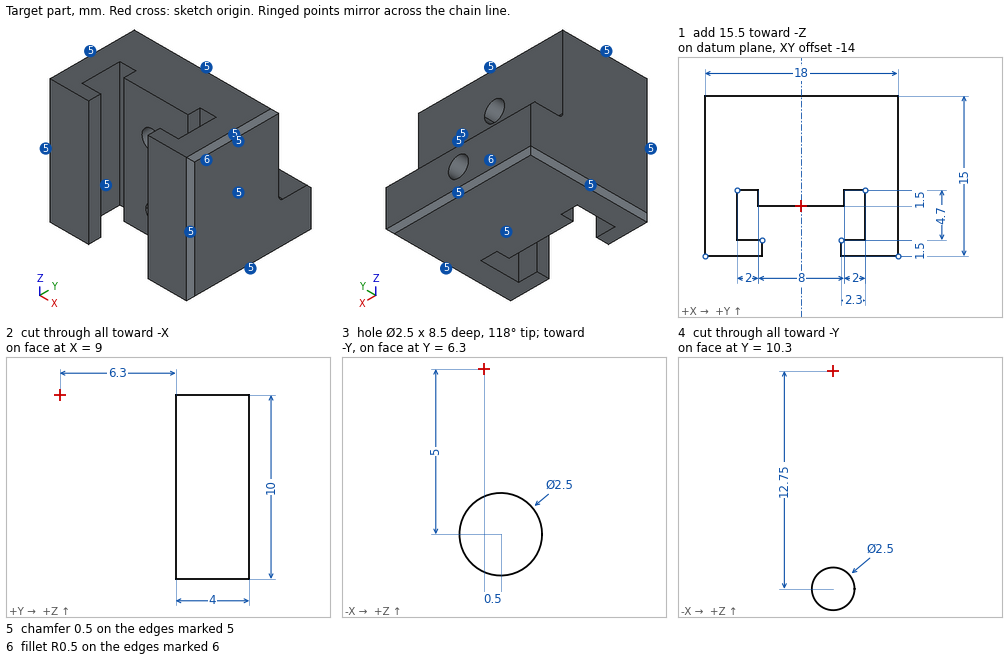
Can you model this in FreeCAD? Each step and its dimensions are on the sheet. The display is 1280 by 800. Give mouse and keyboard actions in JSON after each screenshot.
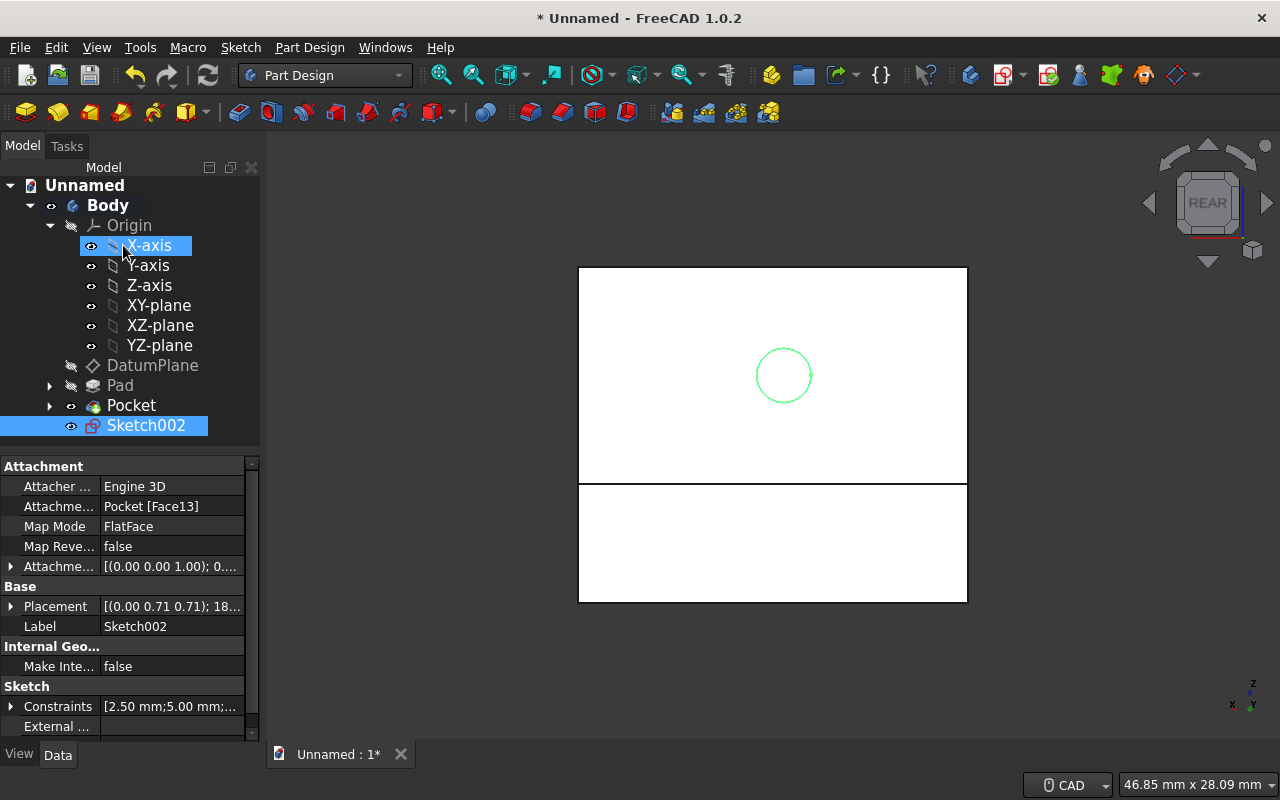
{"action": "left_click", "coordinate": [272, 112]}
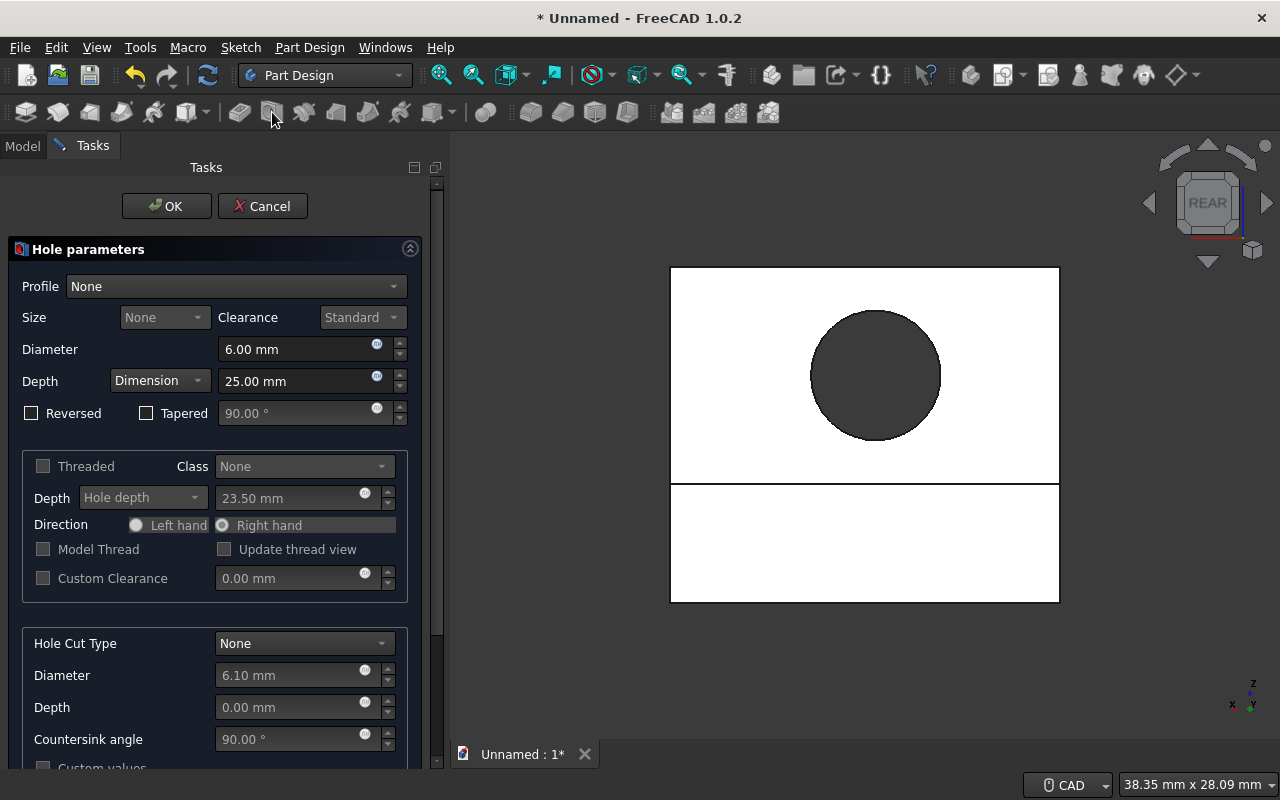
{"action": "triple_click", "coordinate": [305, 349]}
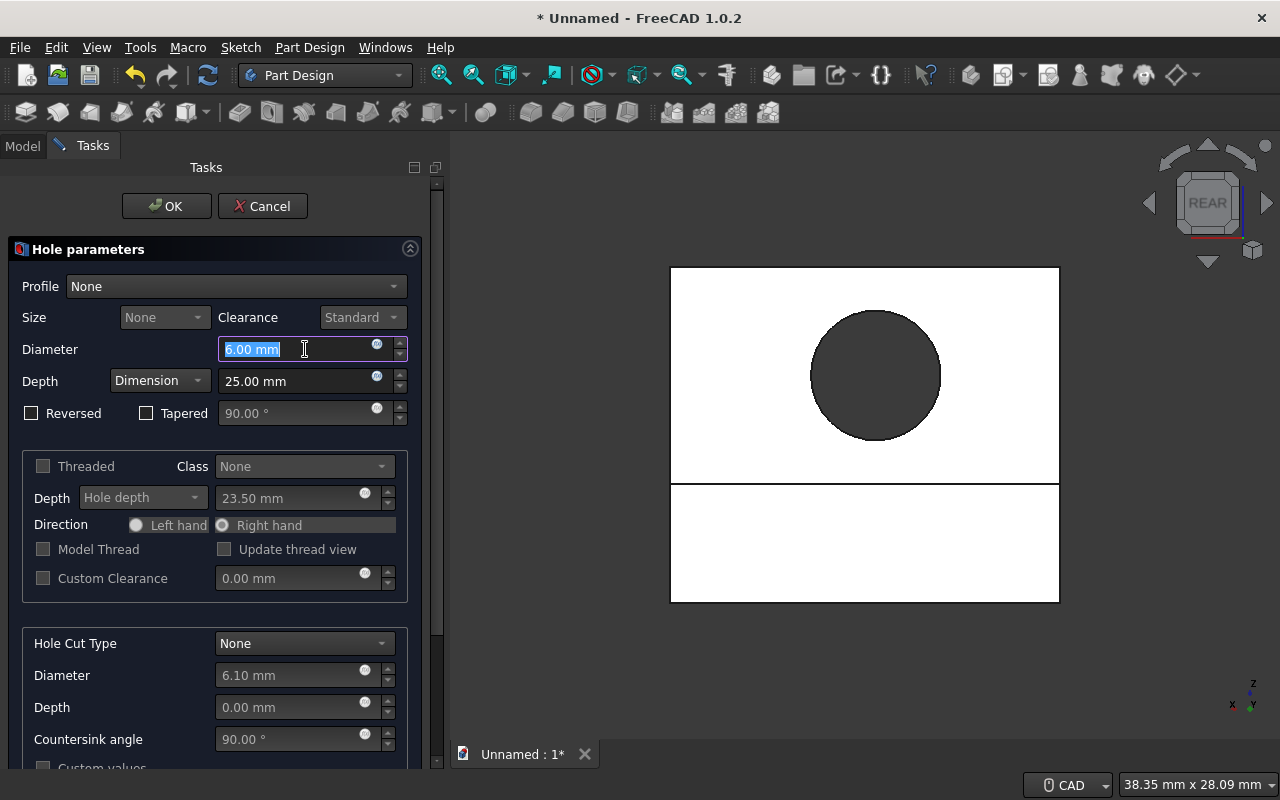
{"action": "type", "text": "2.5"}
{"action": "key", "text": "Tab"}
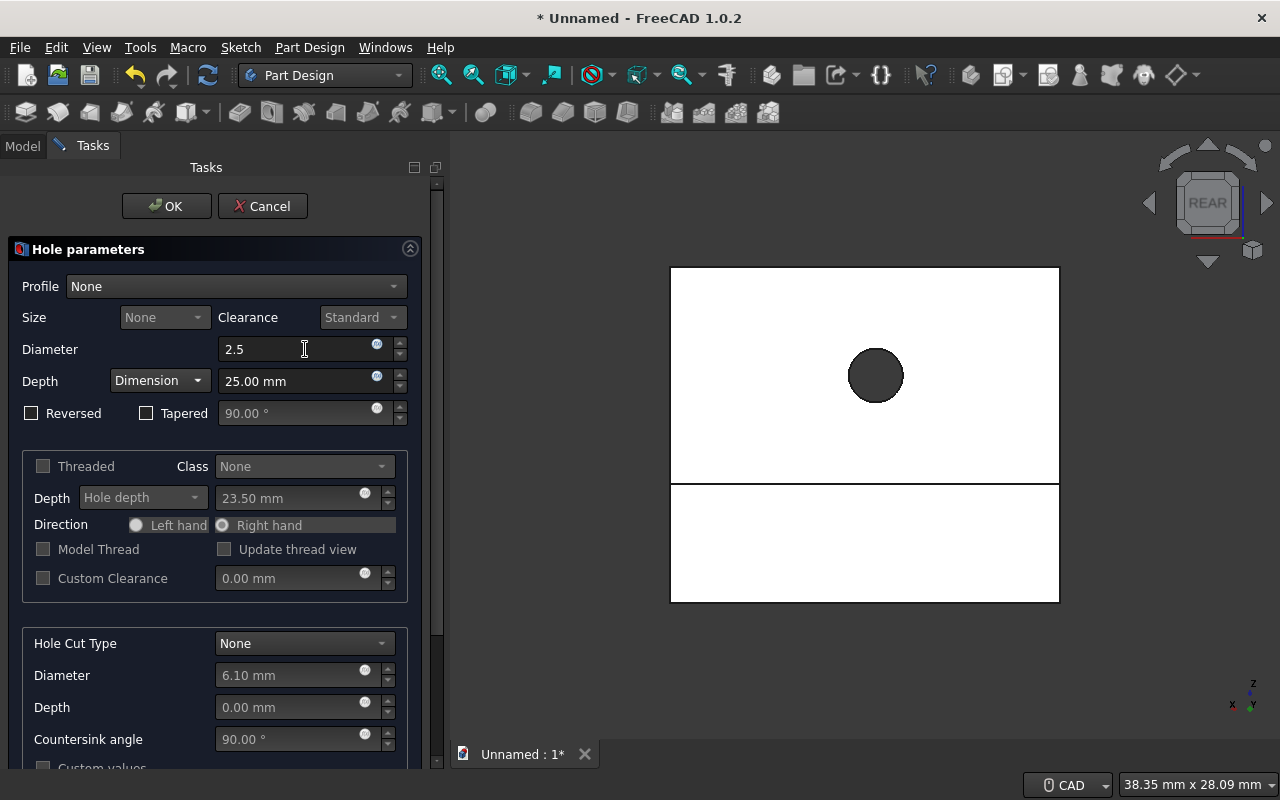
{"action": "triple_click", "coordinate": [305, 381]}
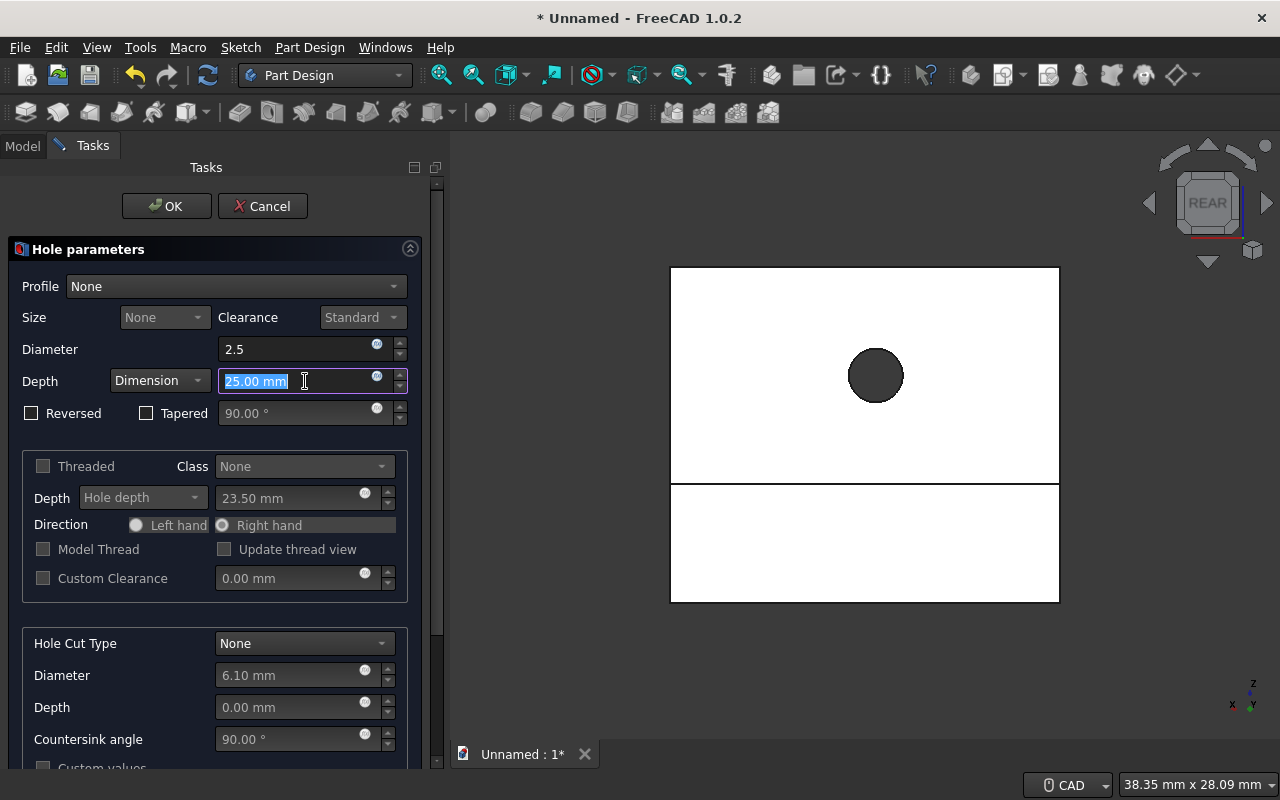
{"action": "type", "text": "8.5"}
{"action": "key", "text": "Tab"}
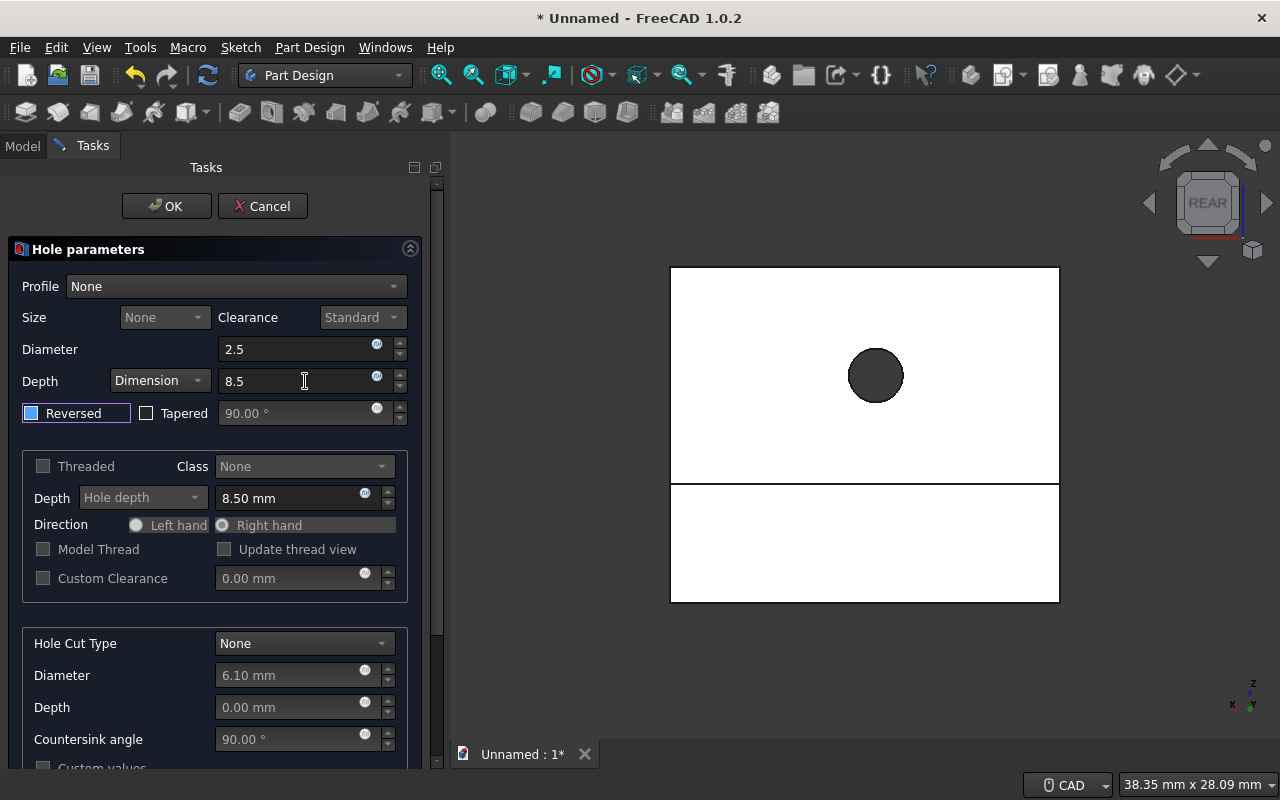
{"action": "left_click", "coordinate": [167, 206]}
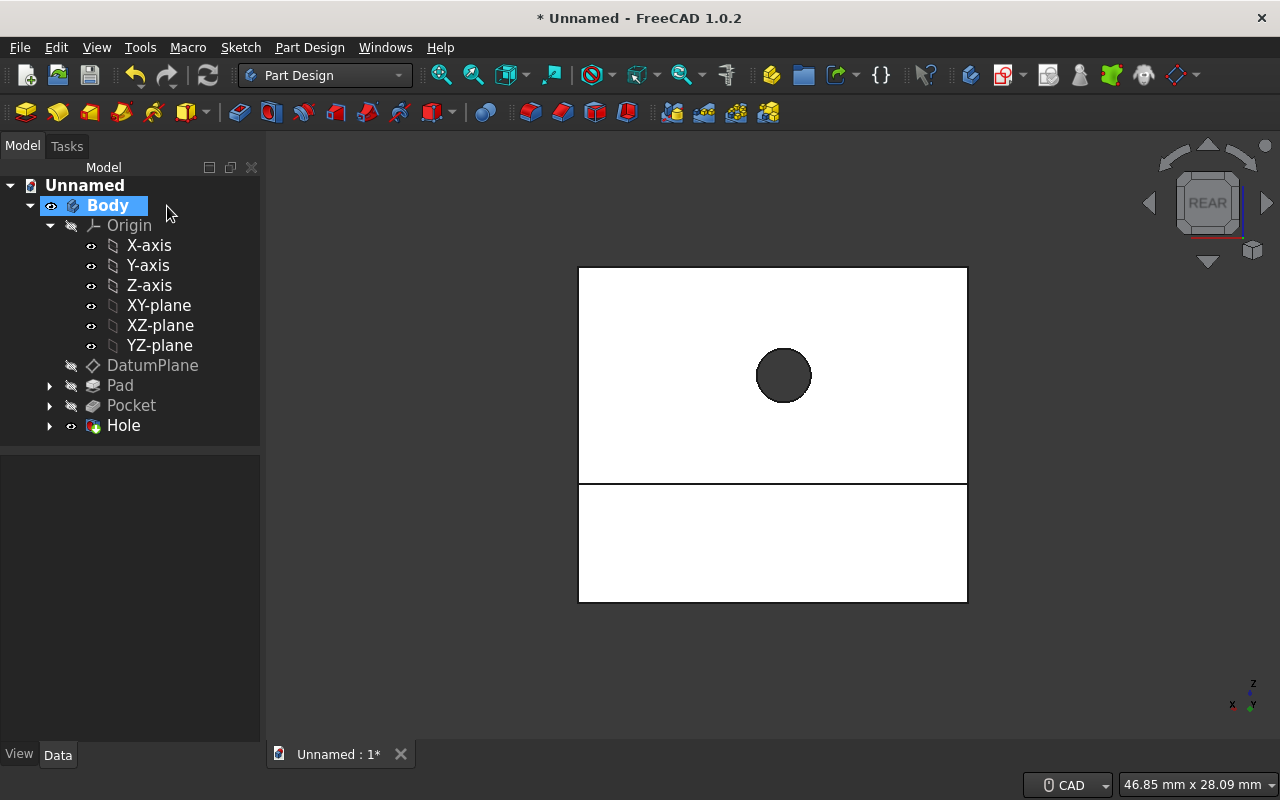
{"action": "left_click", "coordinate": [662, 542]}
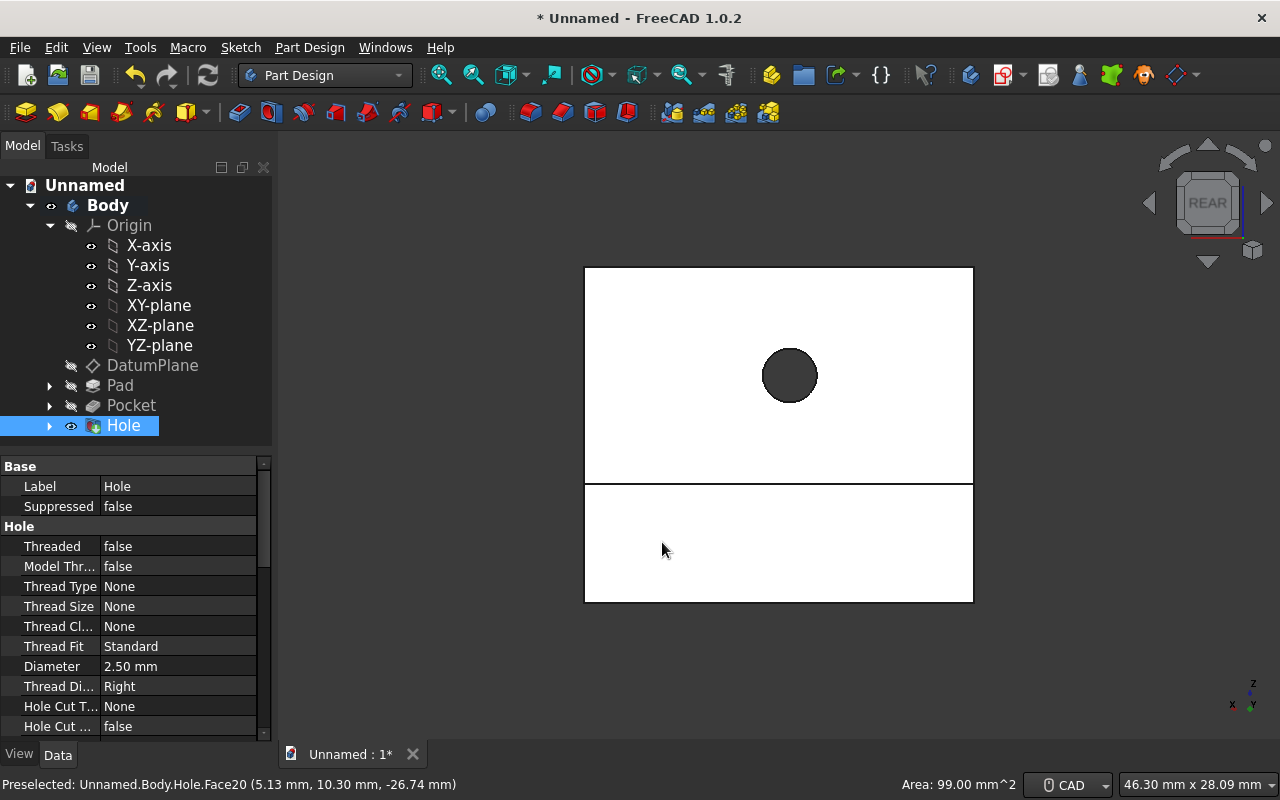
{"action": "left_click", "coordinate": [1004, 76]}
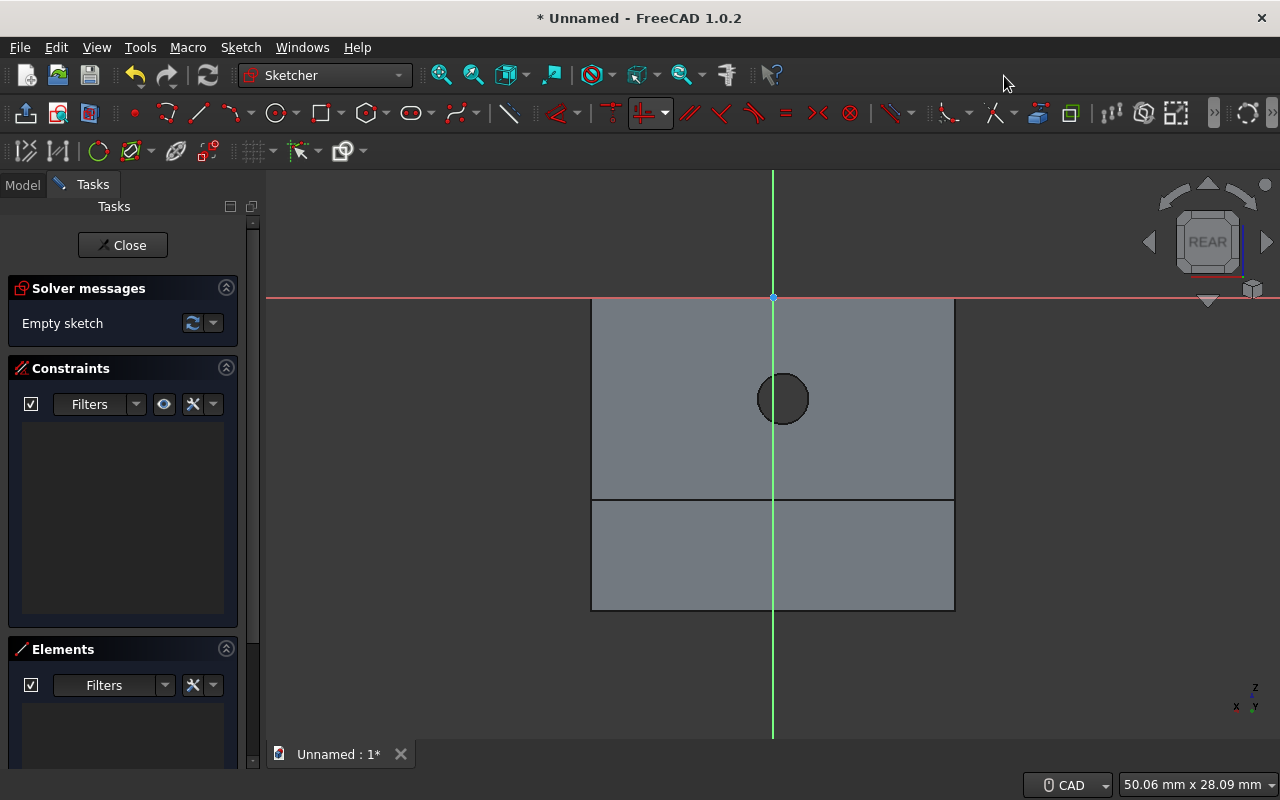
{"action": "scroll", "coordinate": [784, 572], "scroll_direction": "up", "scroll_amount": 10}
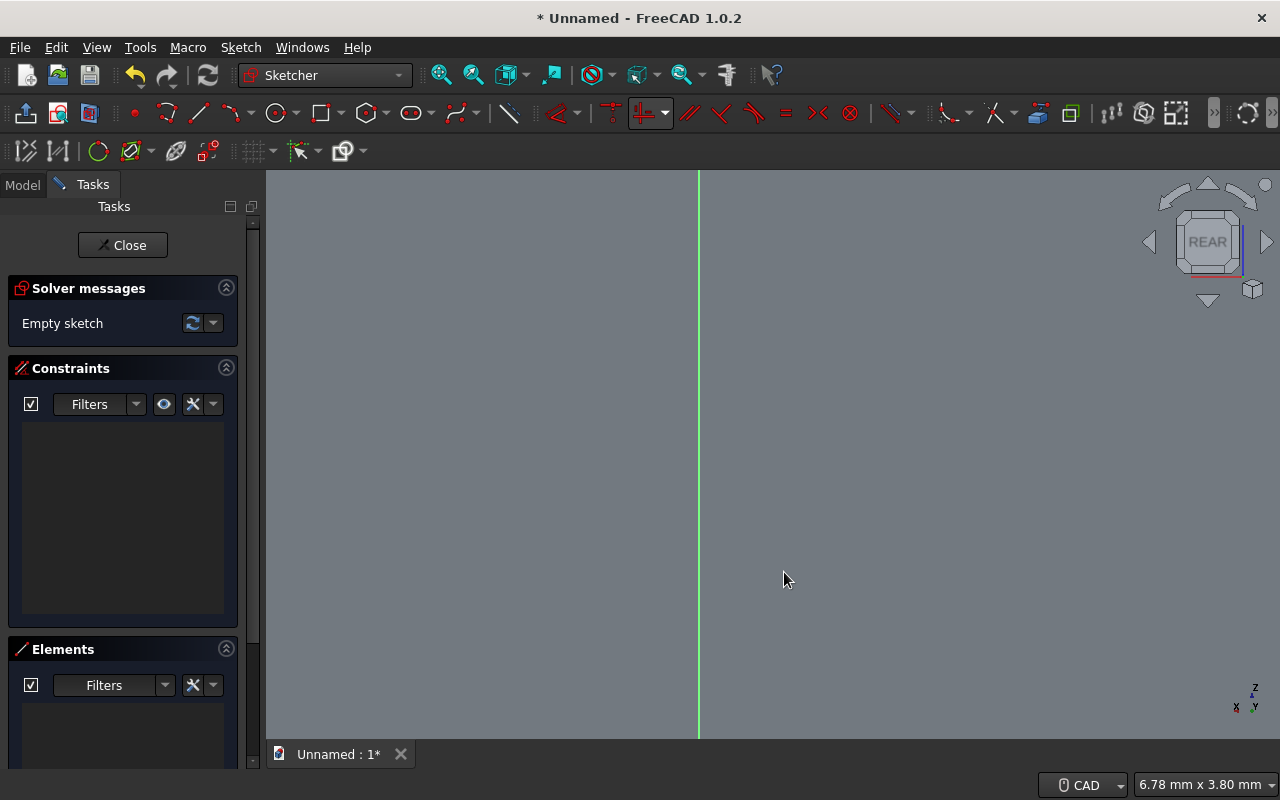
{"action": "left_click", "coordinate": [276, 114]}